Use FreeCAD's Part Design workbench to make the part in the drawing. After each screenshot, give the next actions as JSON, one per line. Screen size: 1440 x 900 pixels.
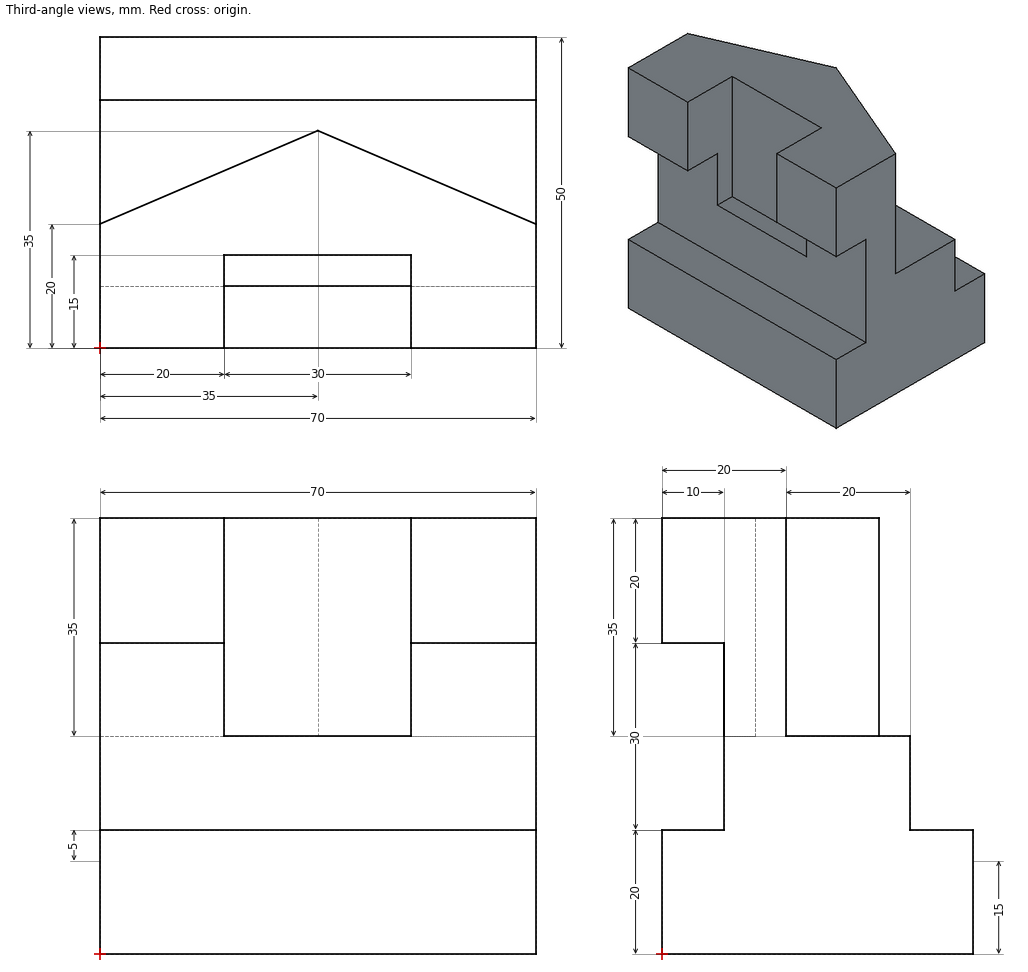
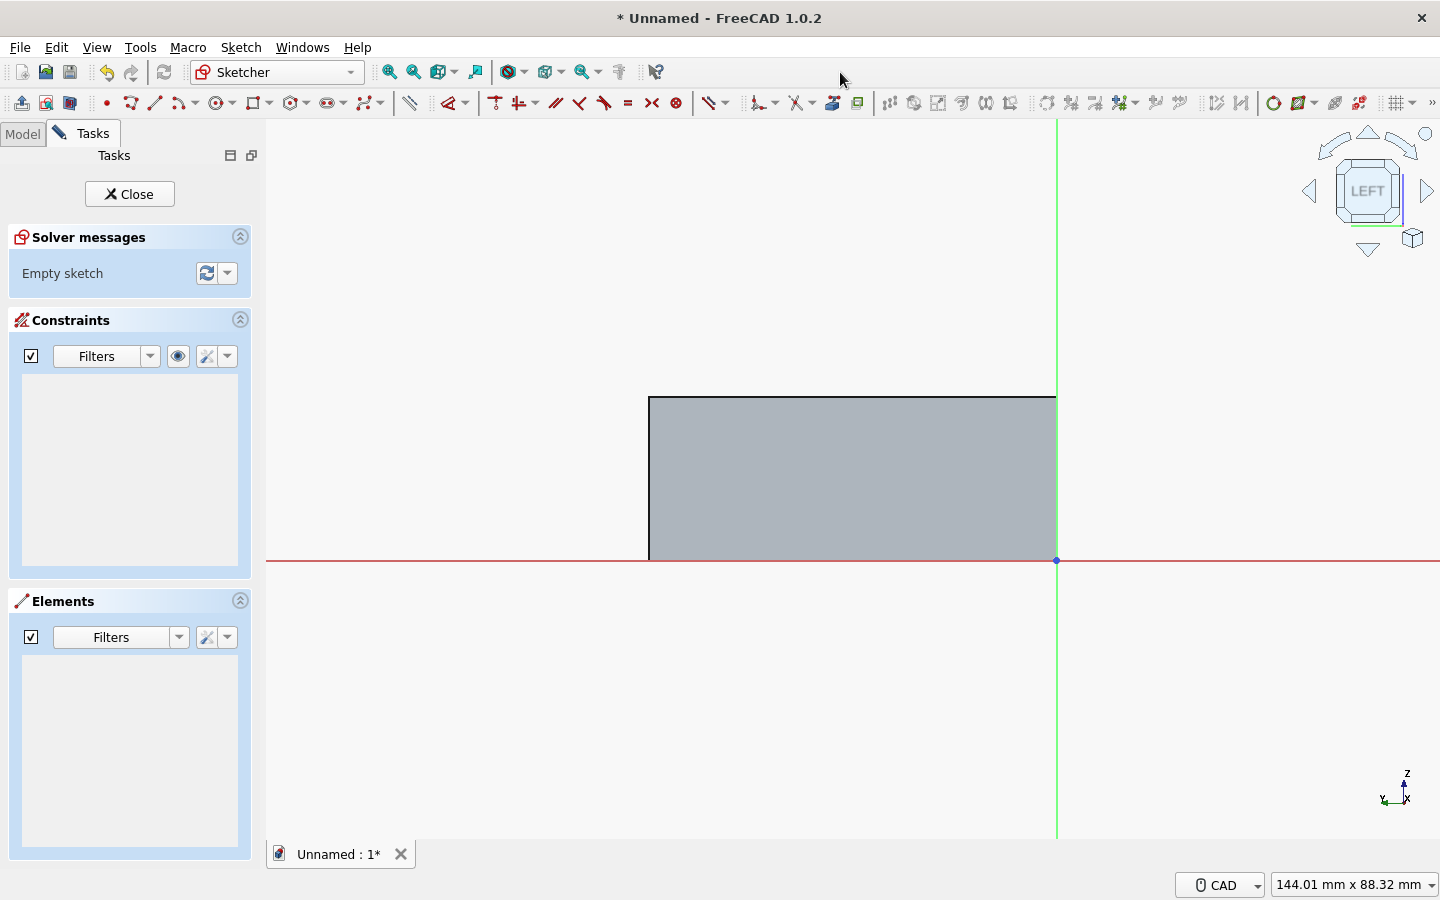
{"action": "scroll", "coordinate": [562, 811], "scroll_direction": "down", "scroll_amount": 2}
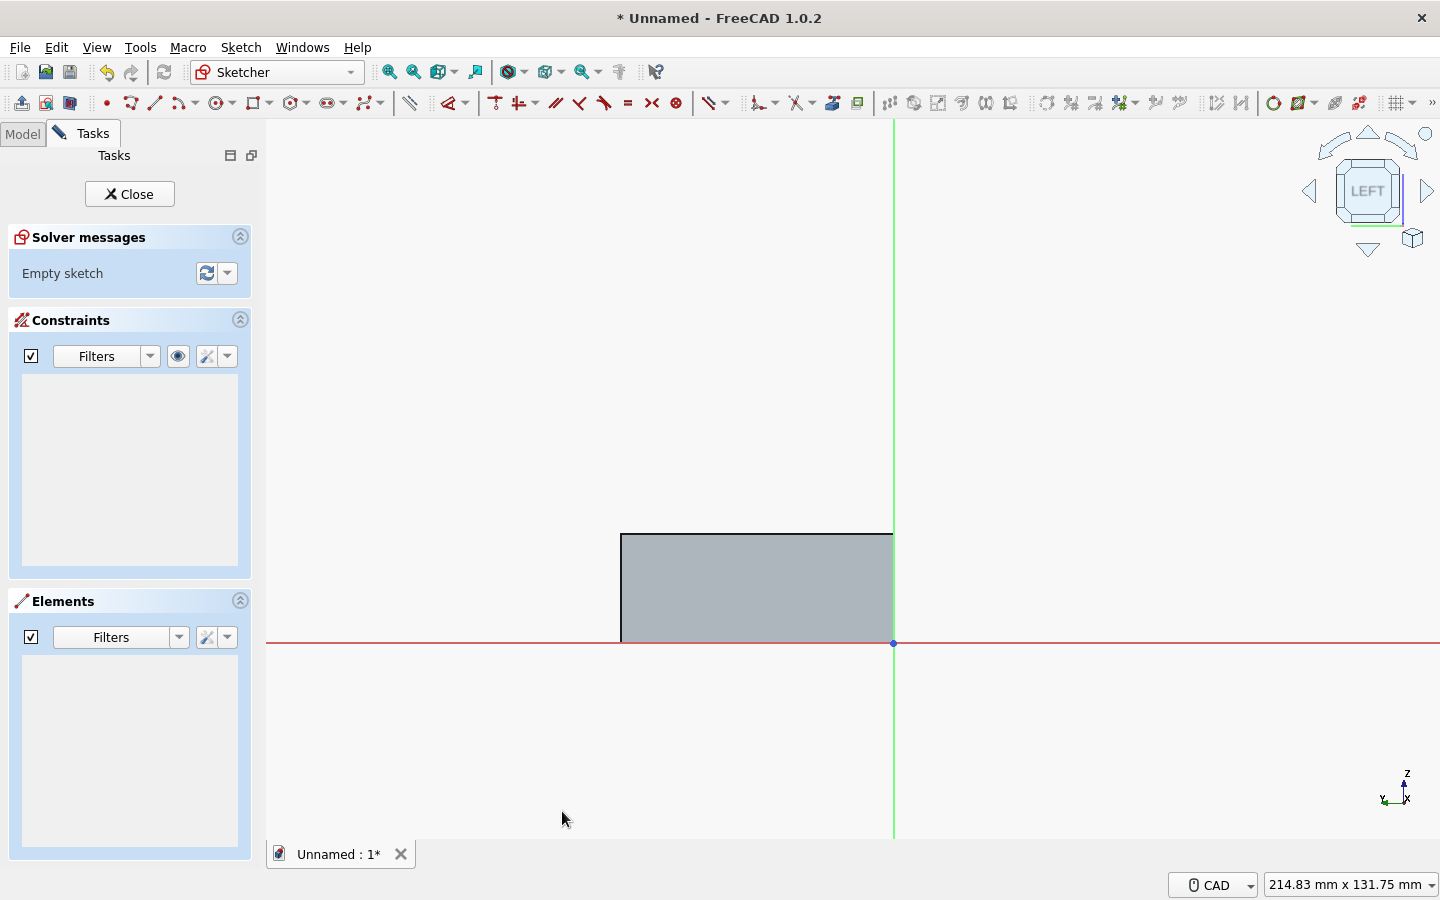
{"action": "left_click", "coordinate": [132, 104]}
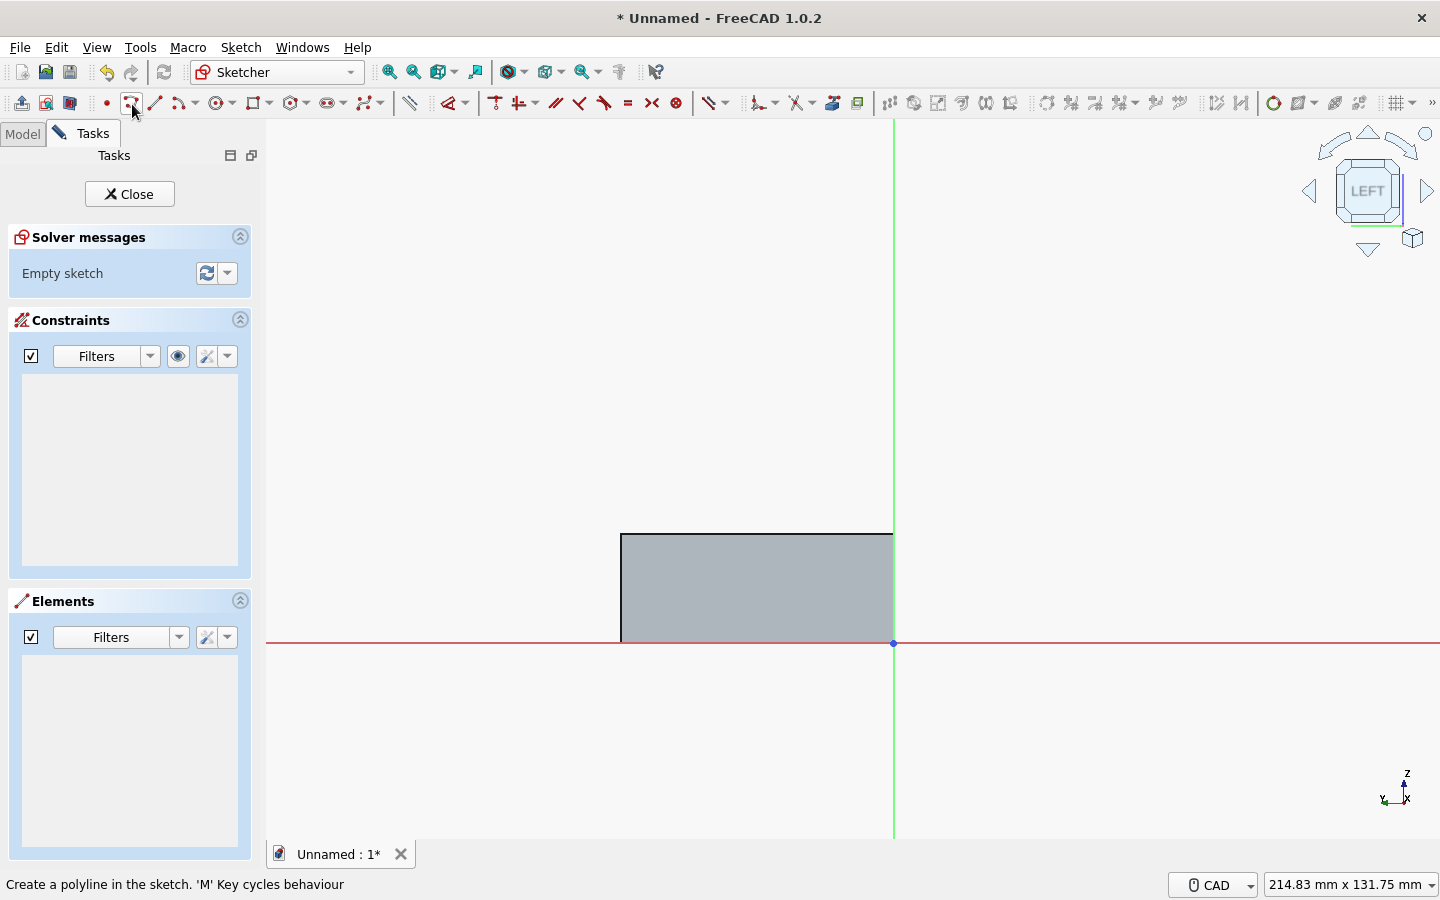
{"action": "left_click", "coordinate": [839, 534]}
{"action": "left_click", "coordinate": [839, 370]}
{"action": "left_click", "coordinate": [894, 370]}
{"action": "left_click", "coordinate": [885, 261]}
{"action": "left_click", "coordinate": [784, 261]}
{"action": "left_click", "coordinate": [784, 452]}
{"action": "left_click", "coordinate": [675, 452]}
{"action": "left_click", "coordinate": [675, 534]}
{"action": "left_click", "coordinate": [839, 535]}
{"action": "key", "text": "Escape"}
{"action": "key", "text": "Escape"}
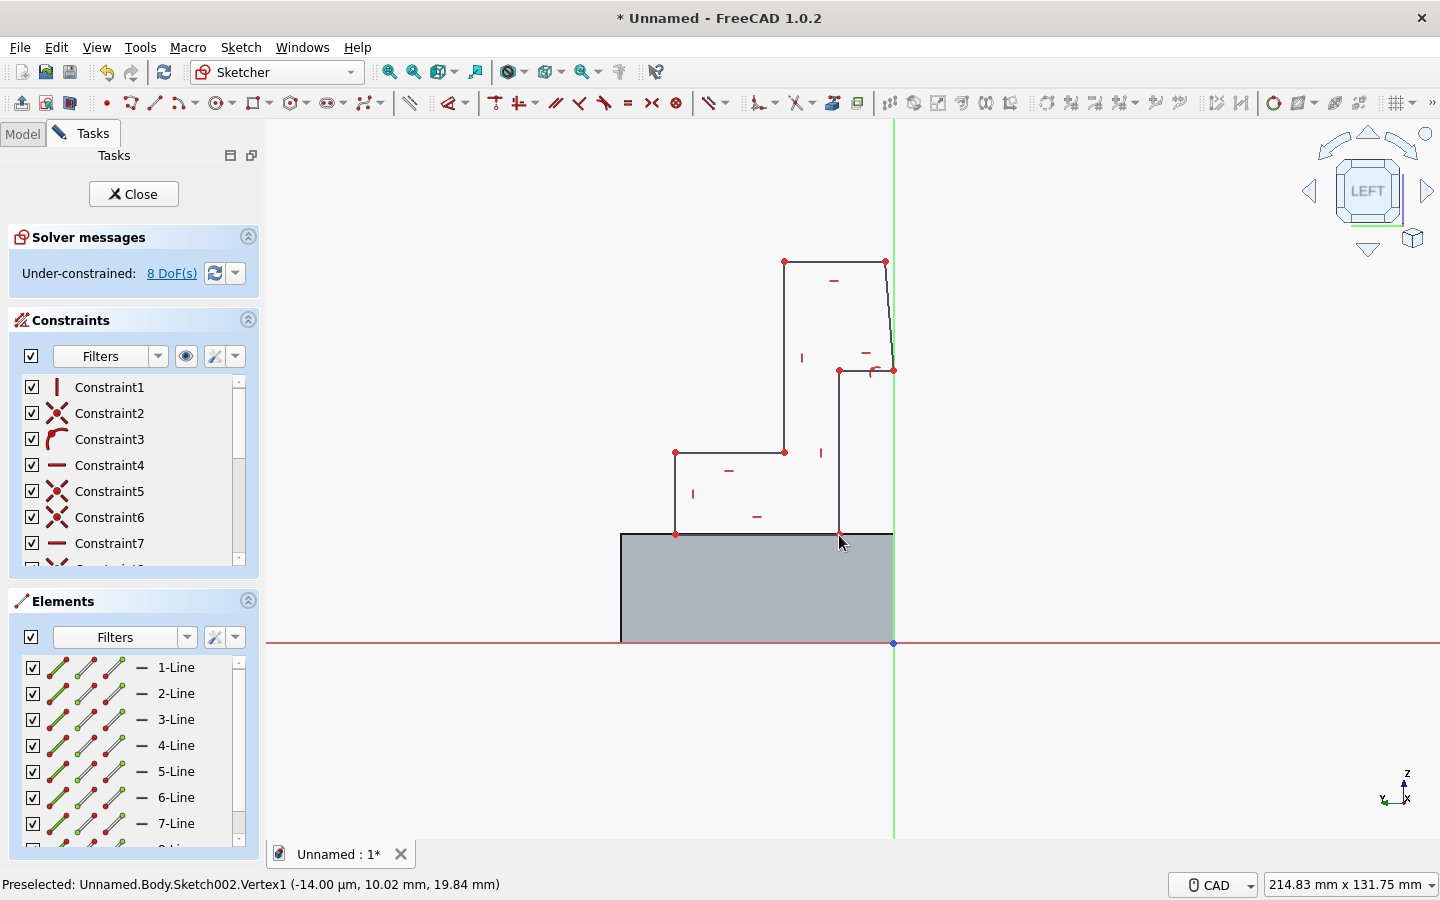
{"action": "left_click", "coordinate": [891, 338]}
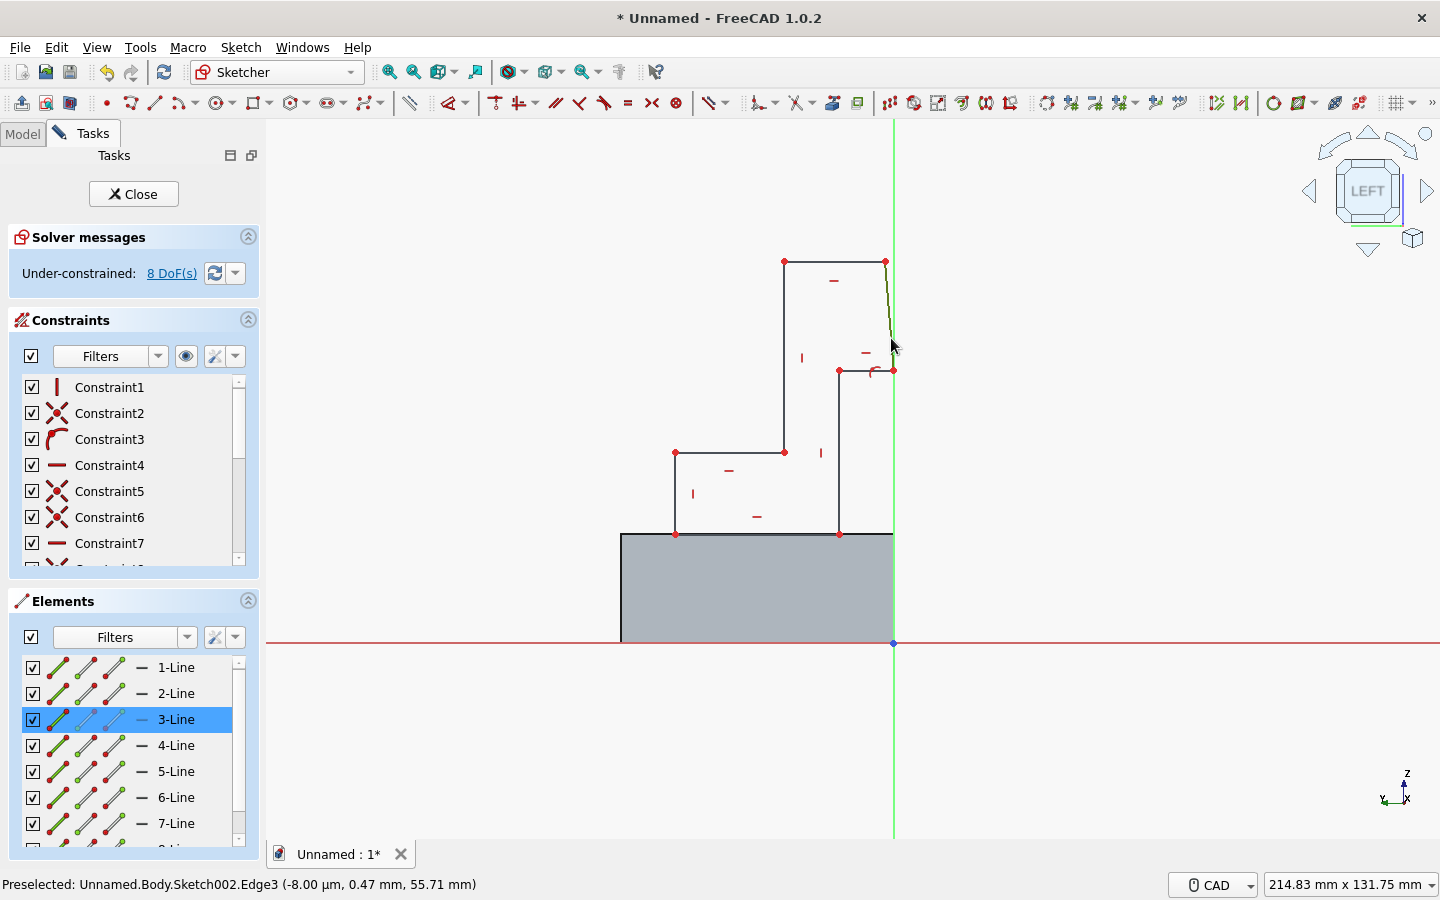
{"action": "left_click", "coordinate": [538, 104]}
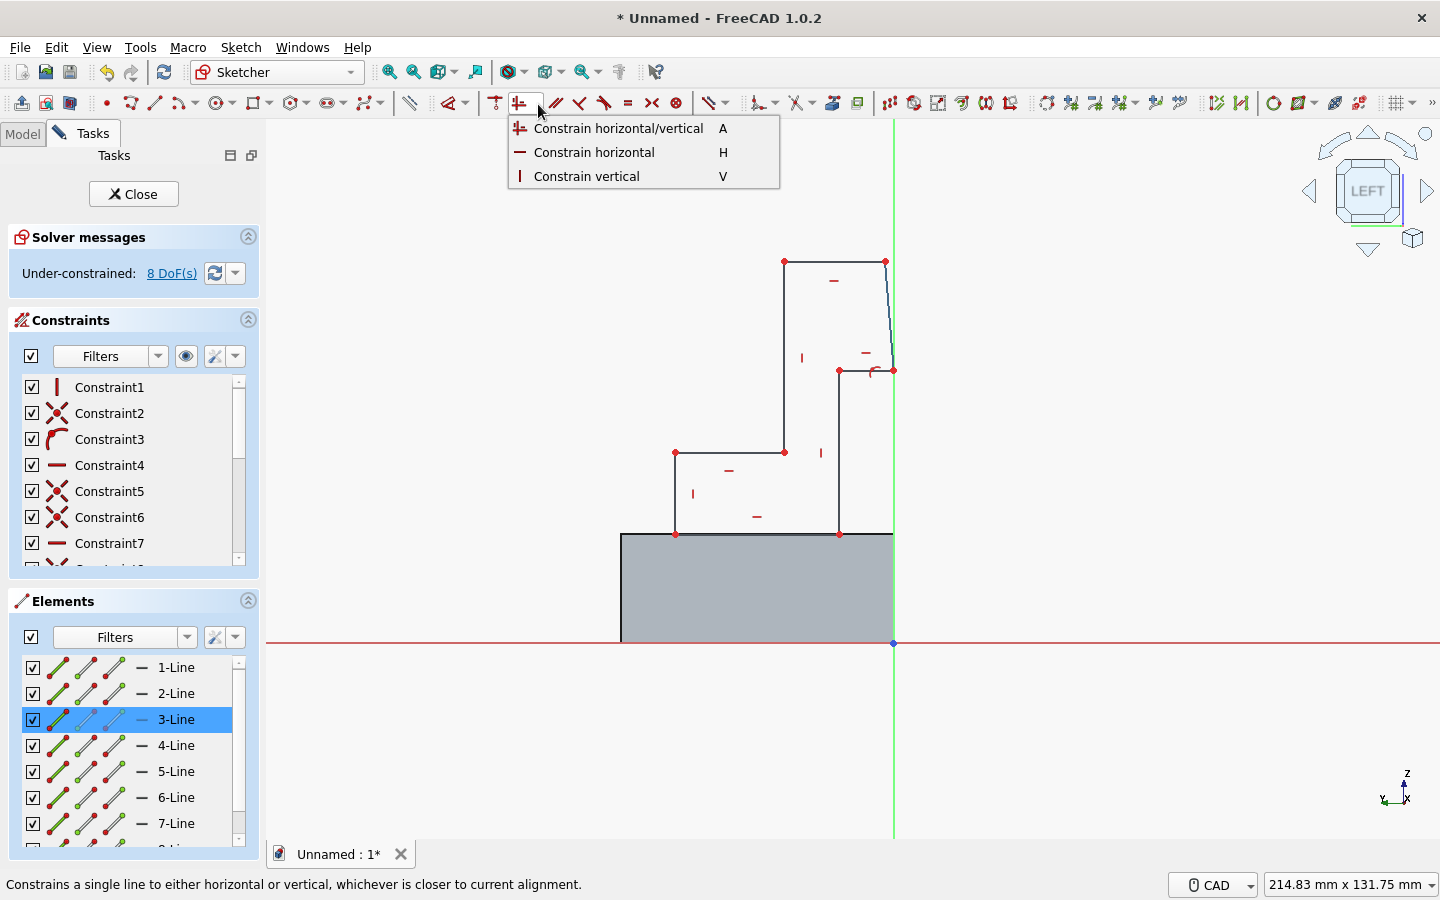
{"action": "left_click", "coordinate": [644, 176]}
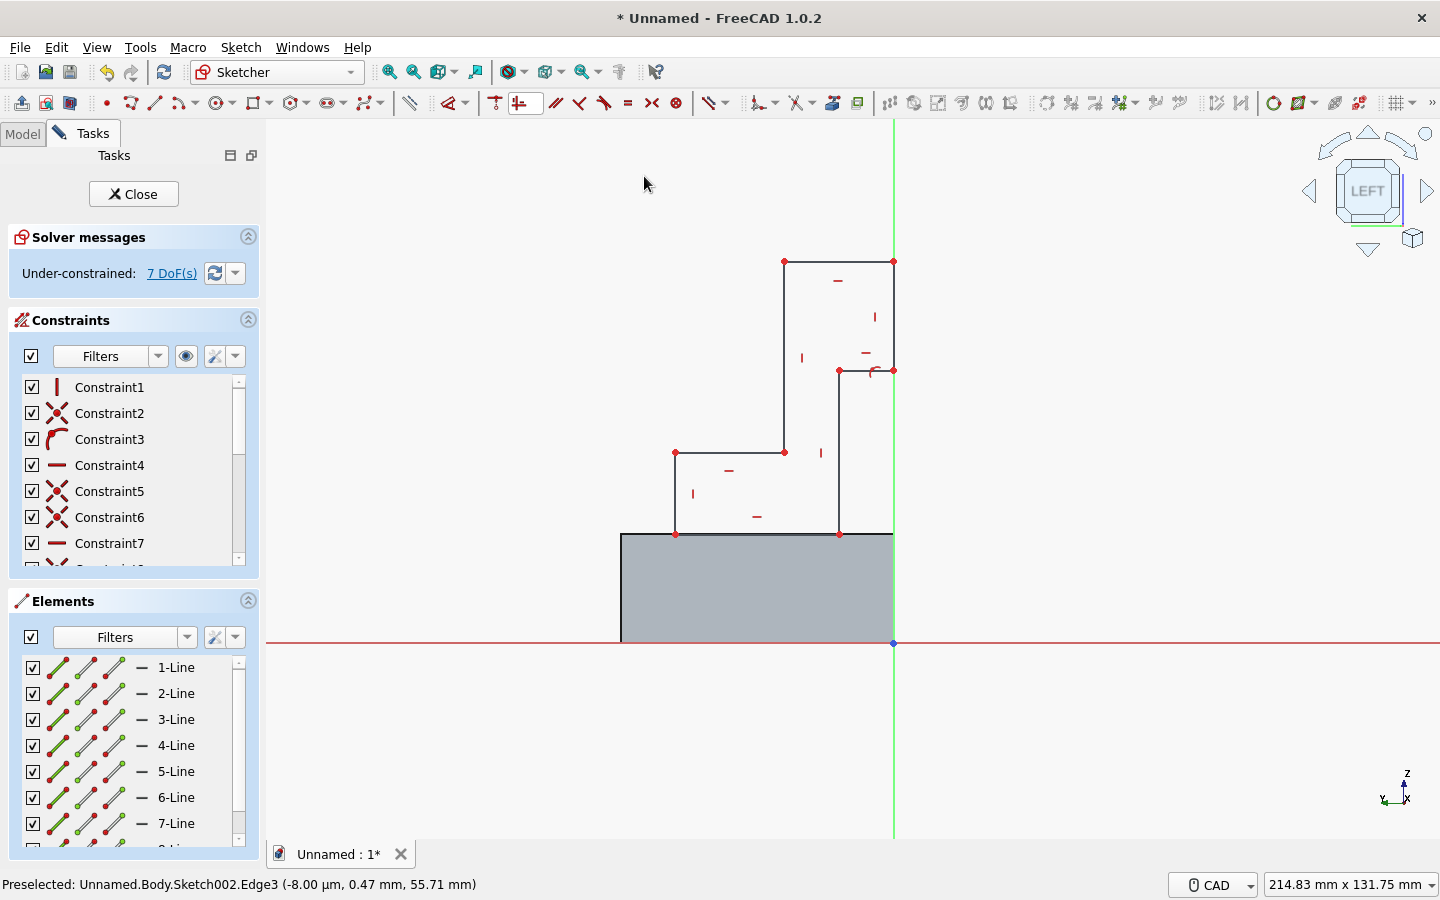
{"action": "left_click", "coordinate": [448, 104]}